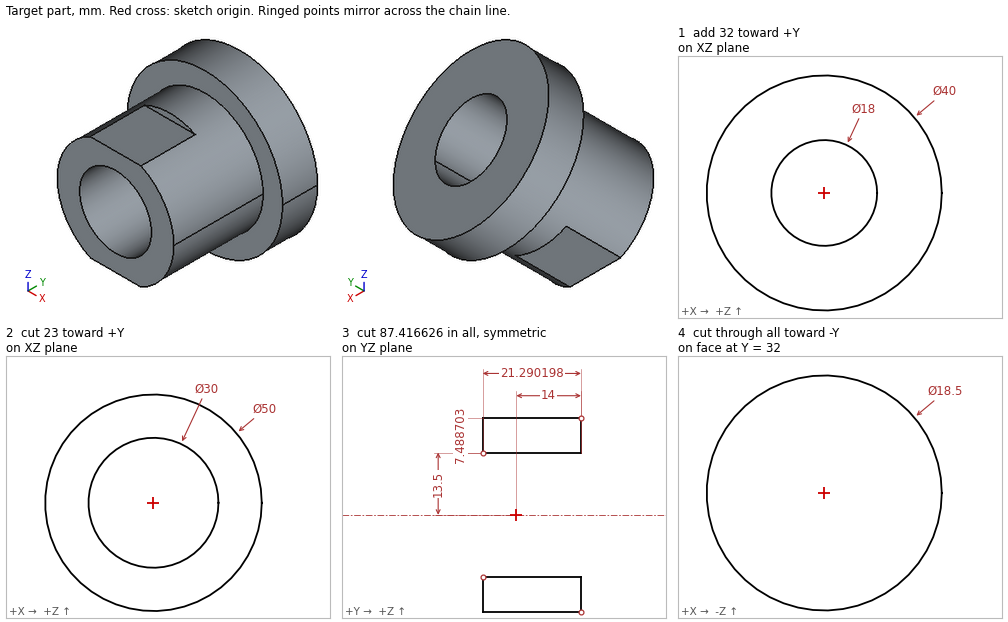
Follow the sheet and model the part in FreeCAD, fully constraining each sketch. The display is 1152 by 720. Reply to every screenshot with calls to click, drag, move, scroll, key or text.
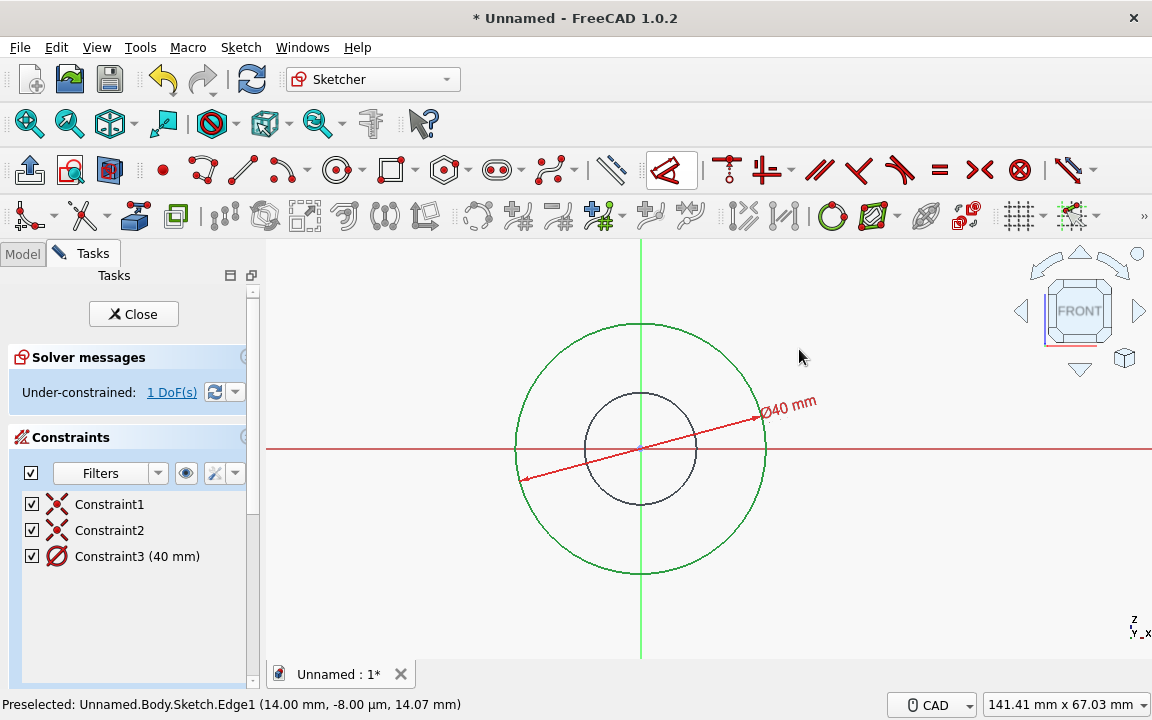
click(680, 409)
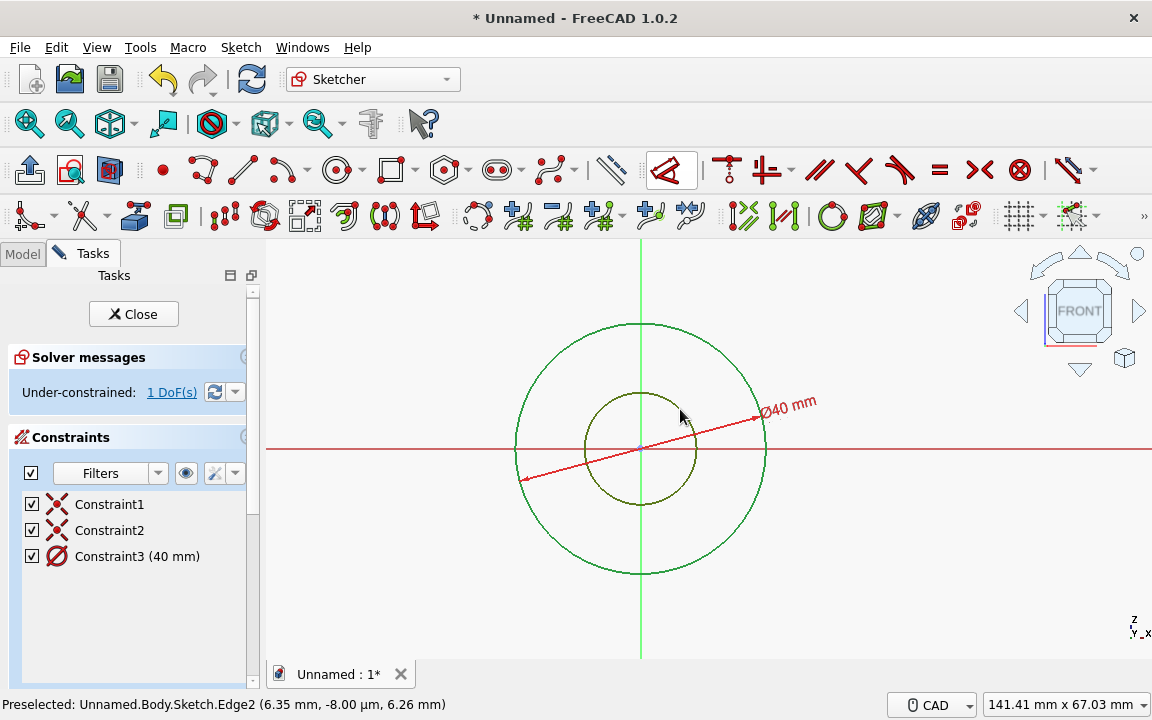
click(692, 170)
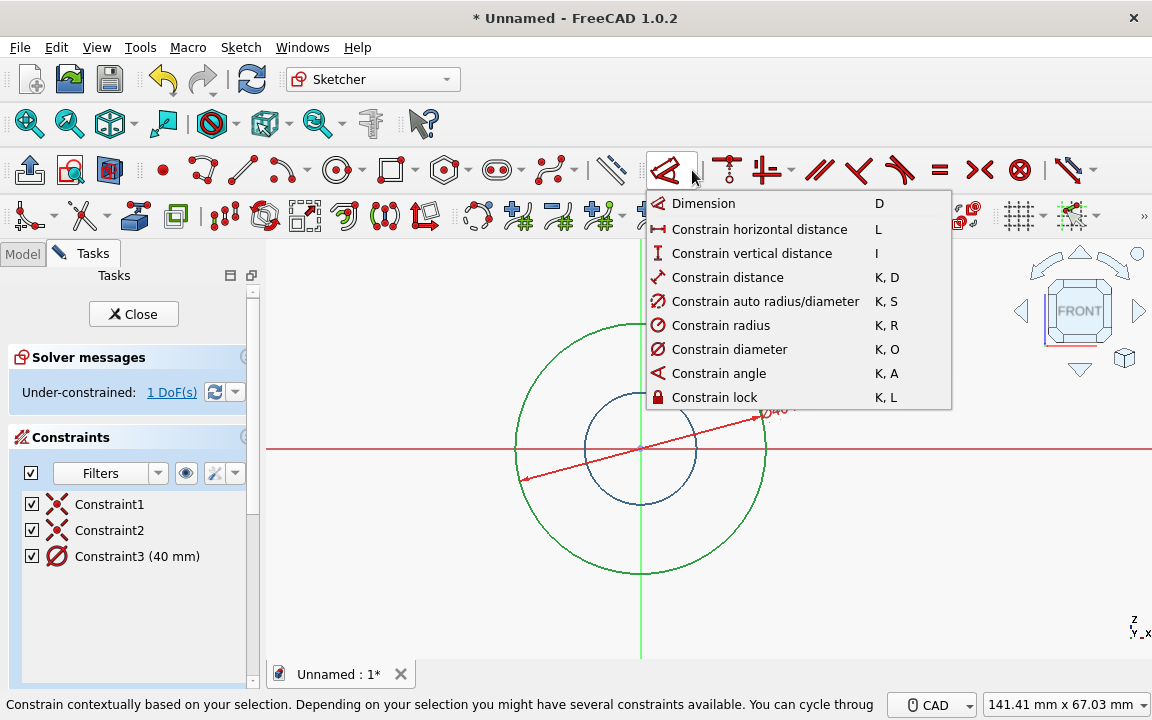
click(799, 349)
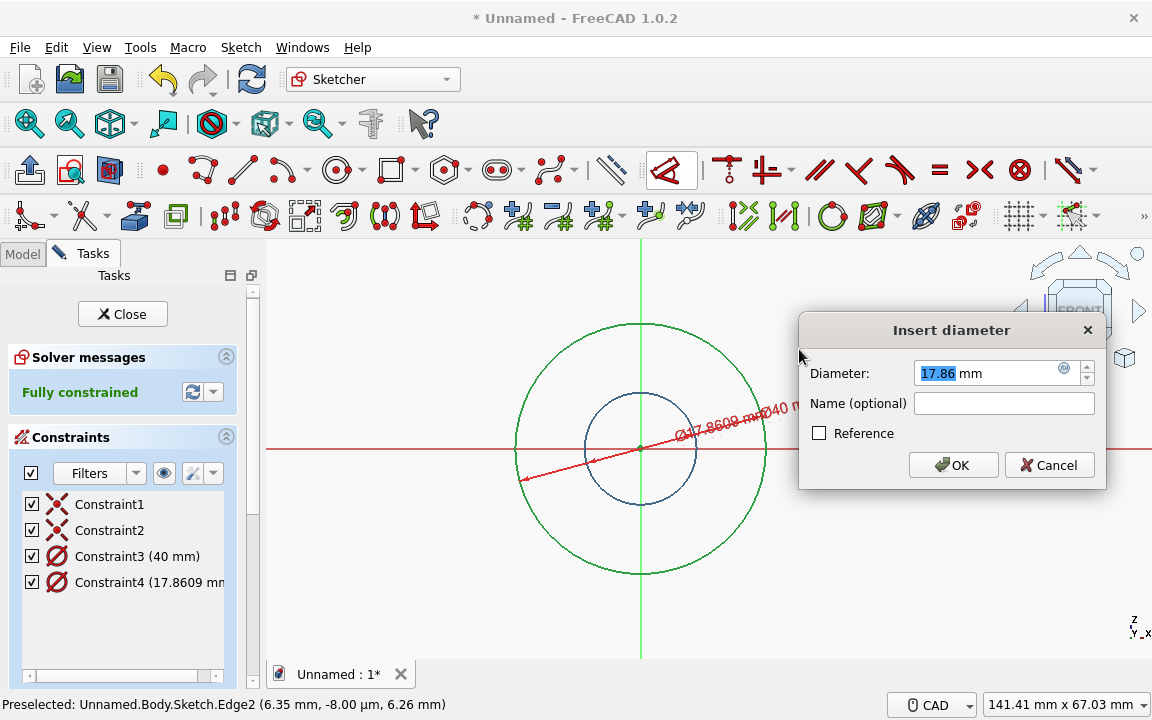
text(18)
key(Return)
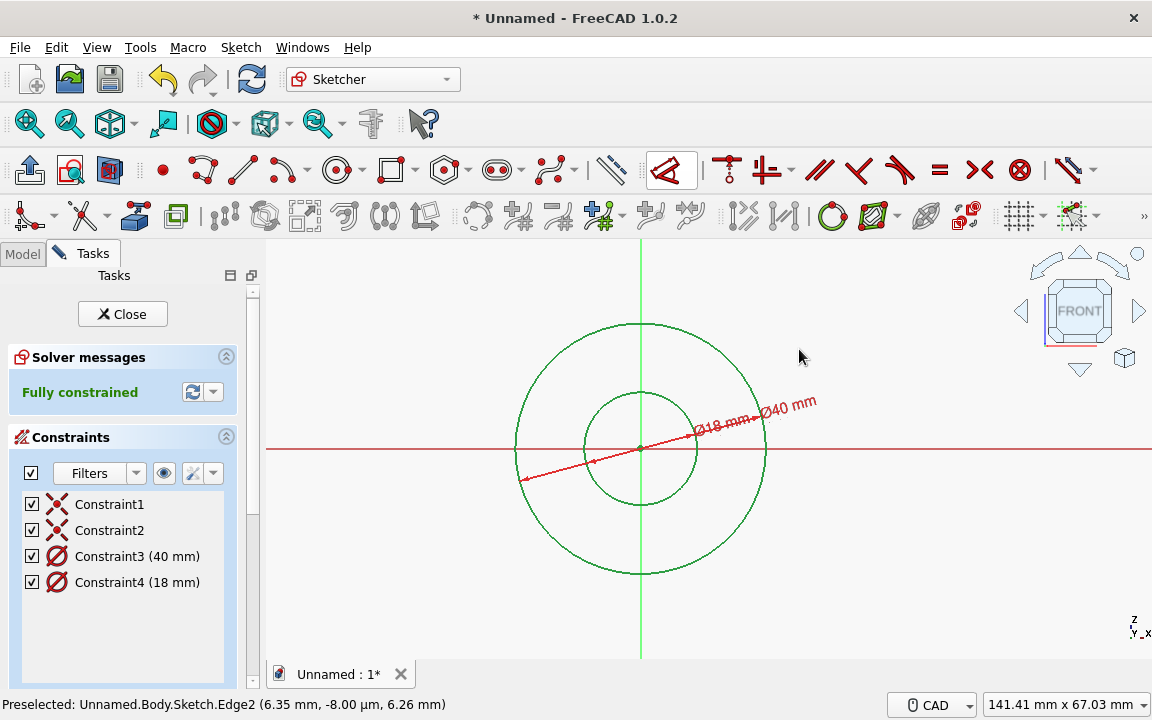
click(123, 314)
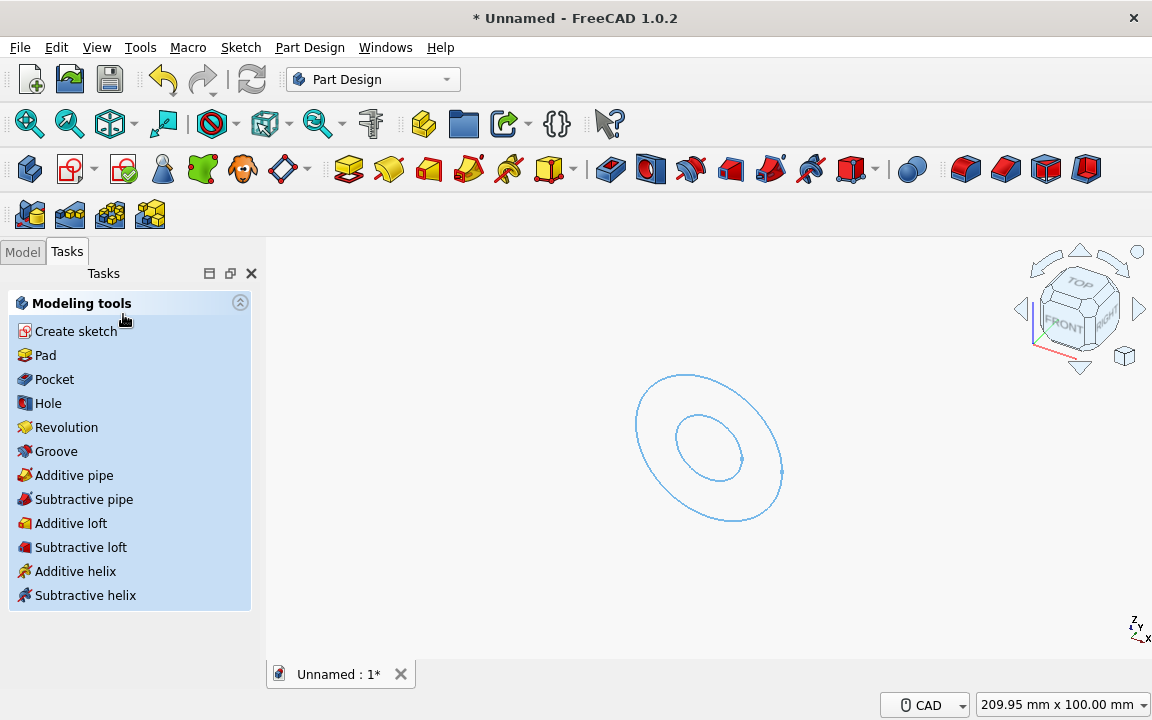
click(350, 170)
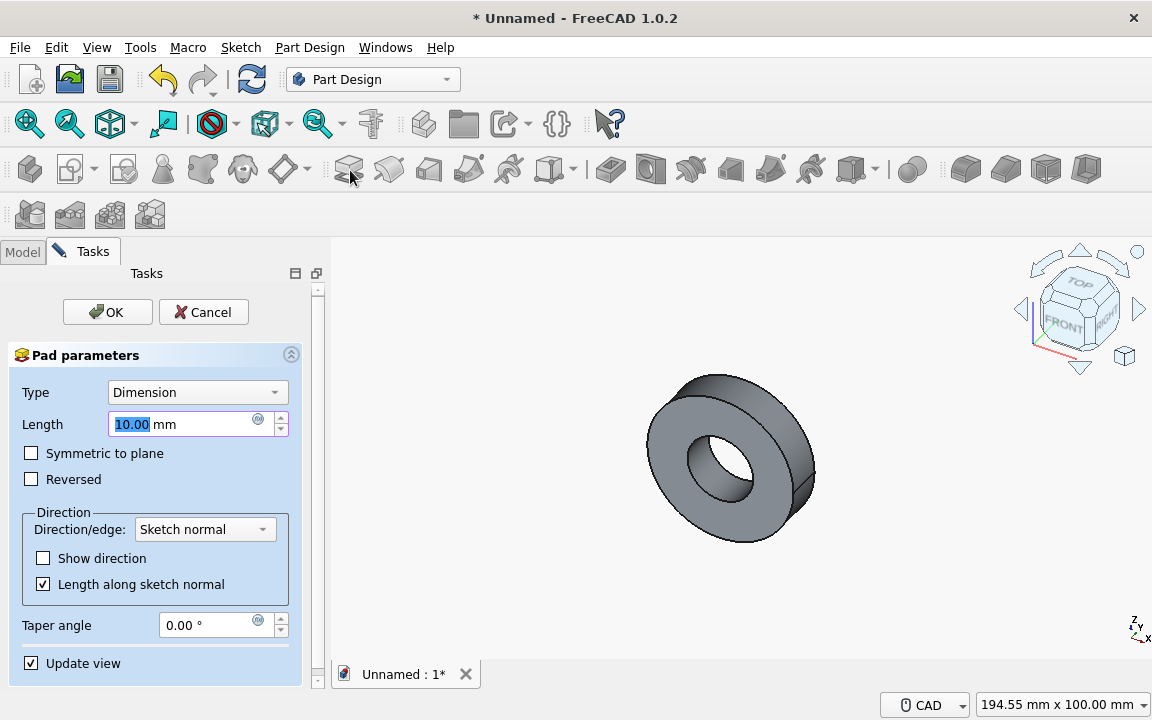
text(32)
key(Tab)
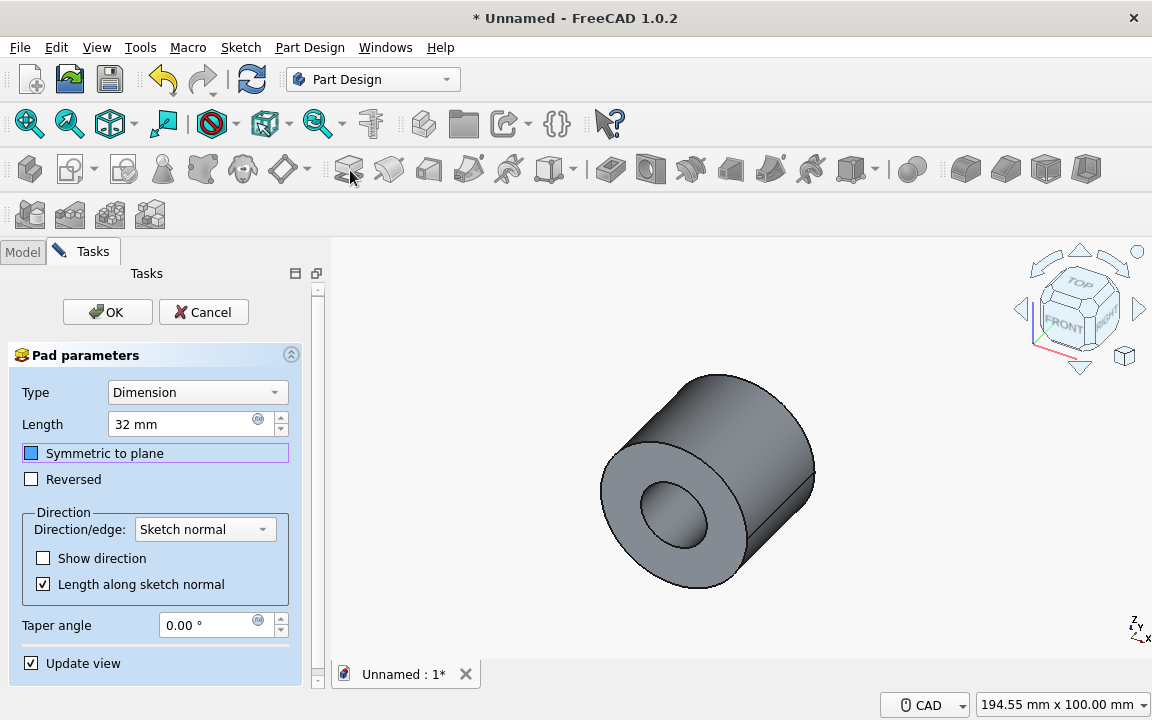
click(30, 479)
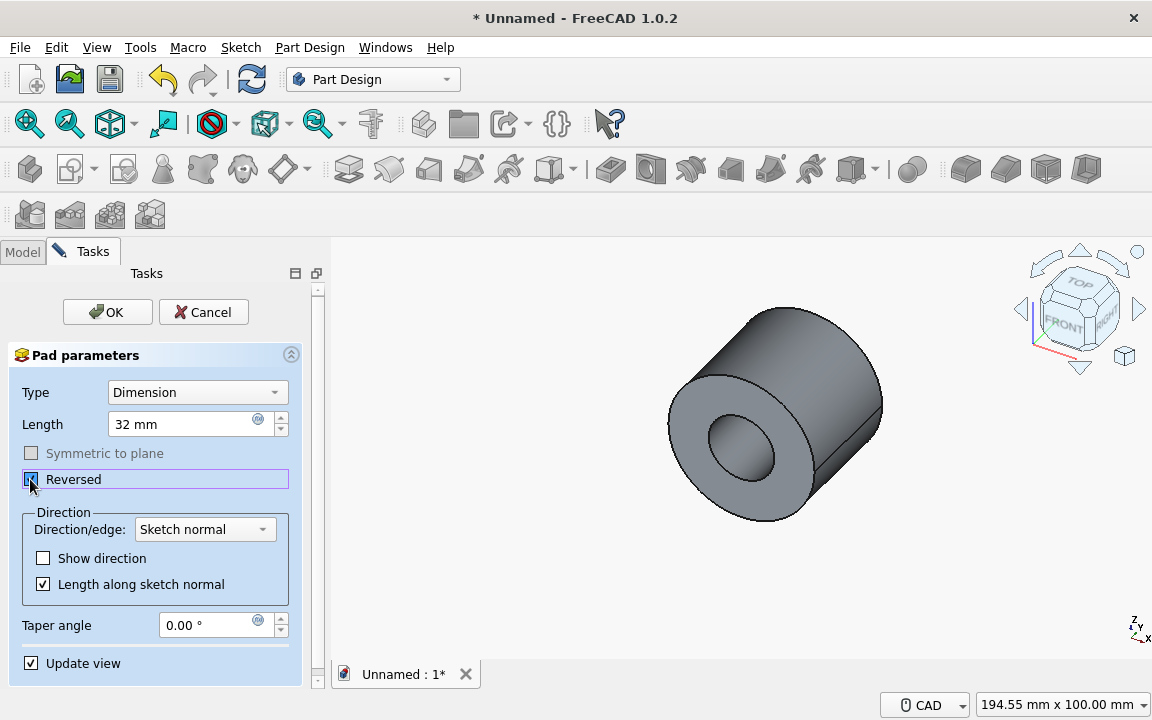
click(108, 312)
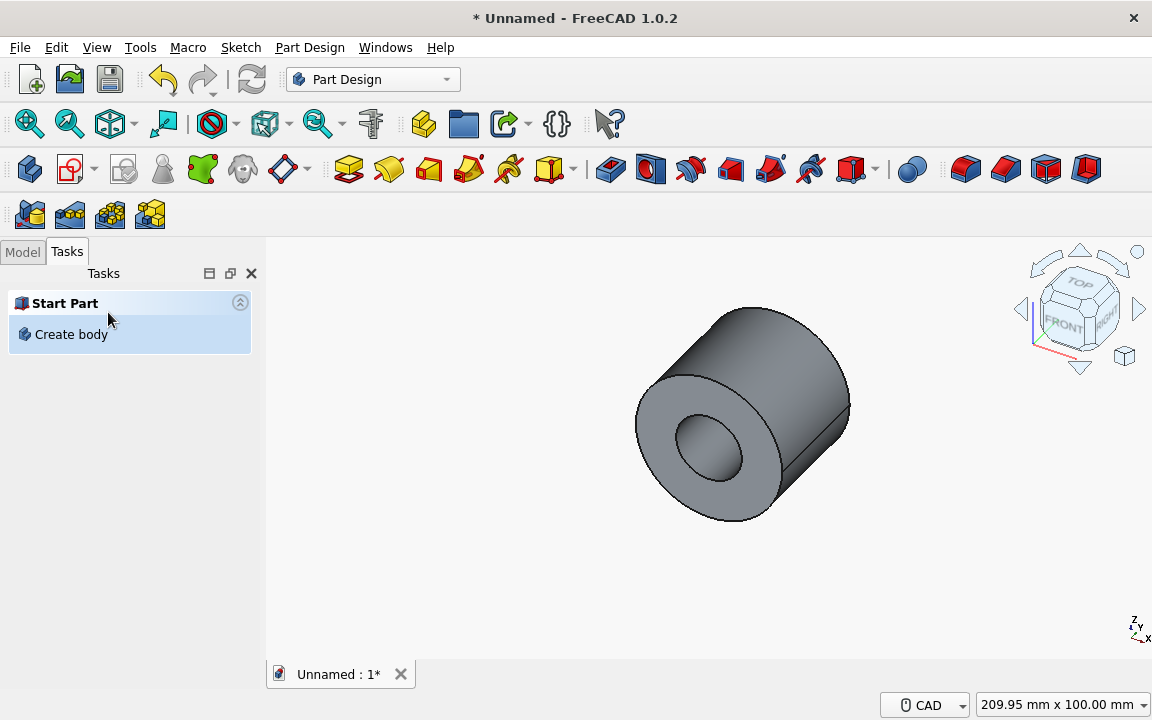
click(70, 170)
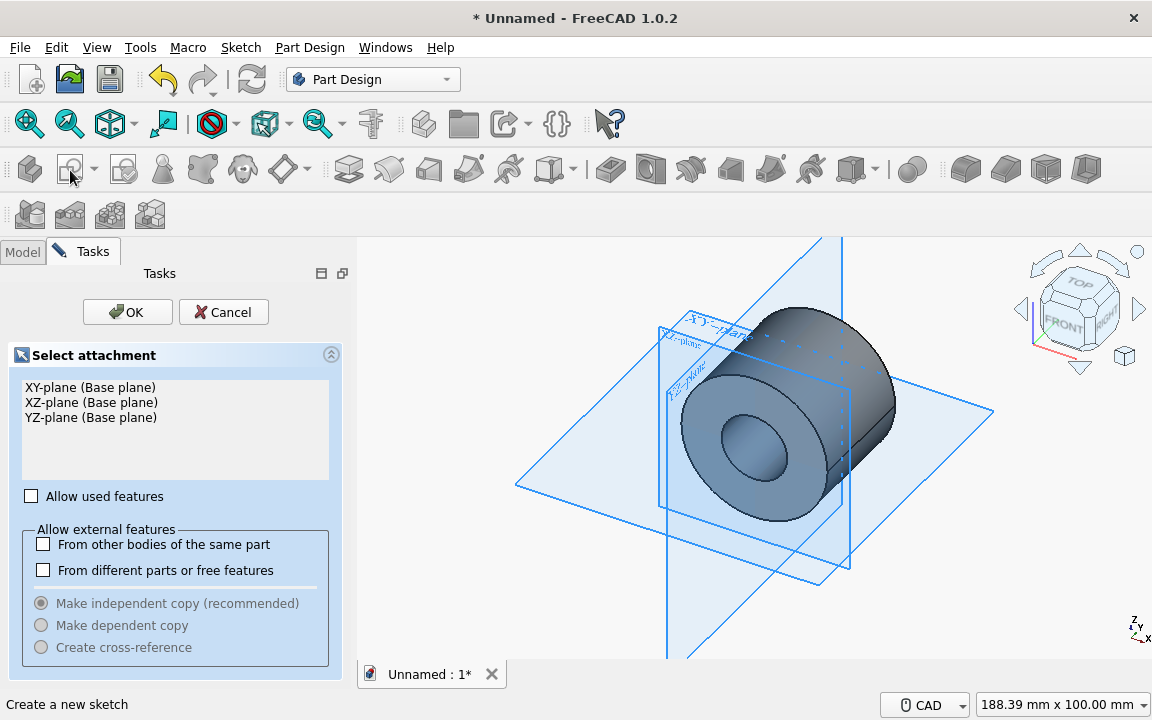
click(82, 402)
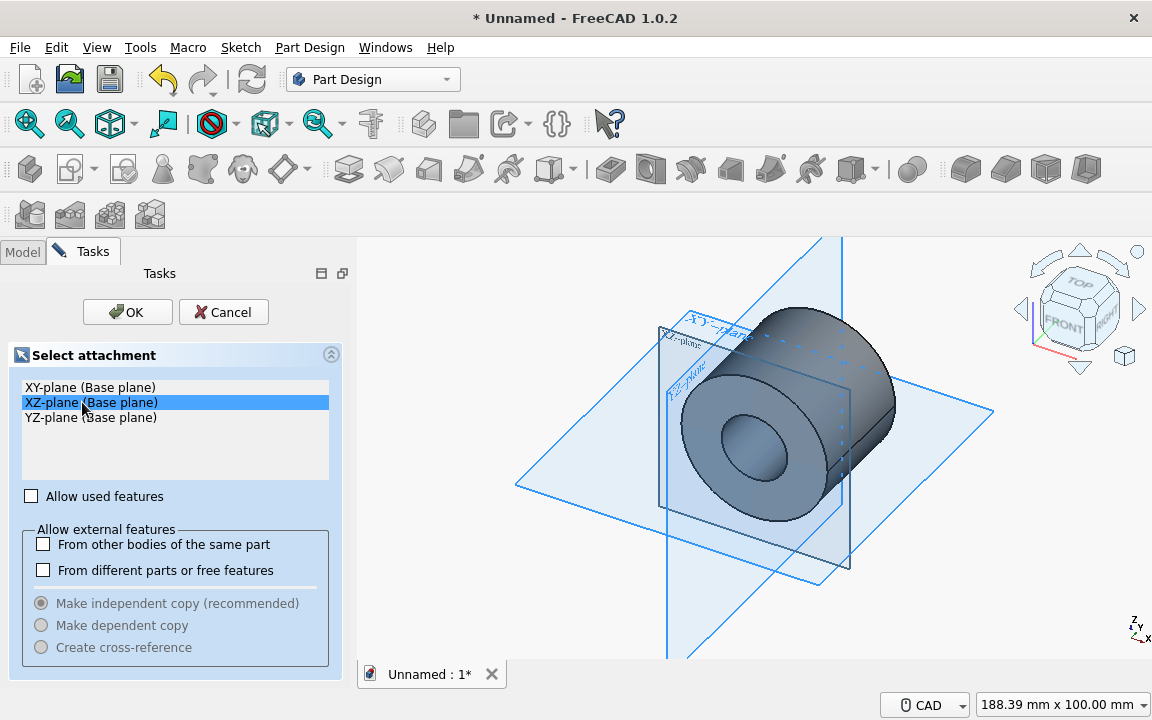
click(128, 312)